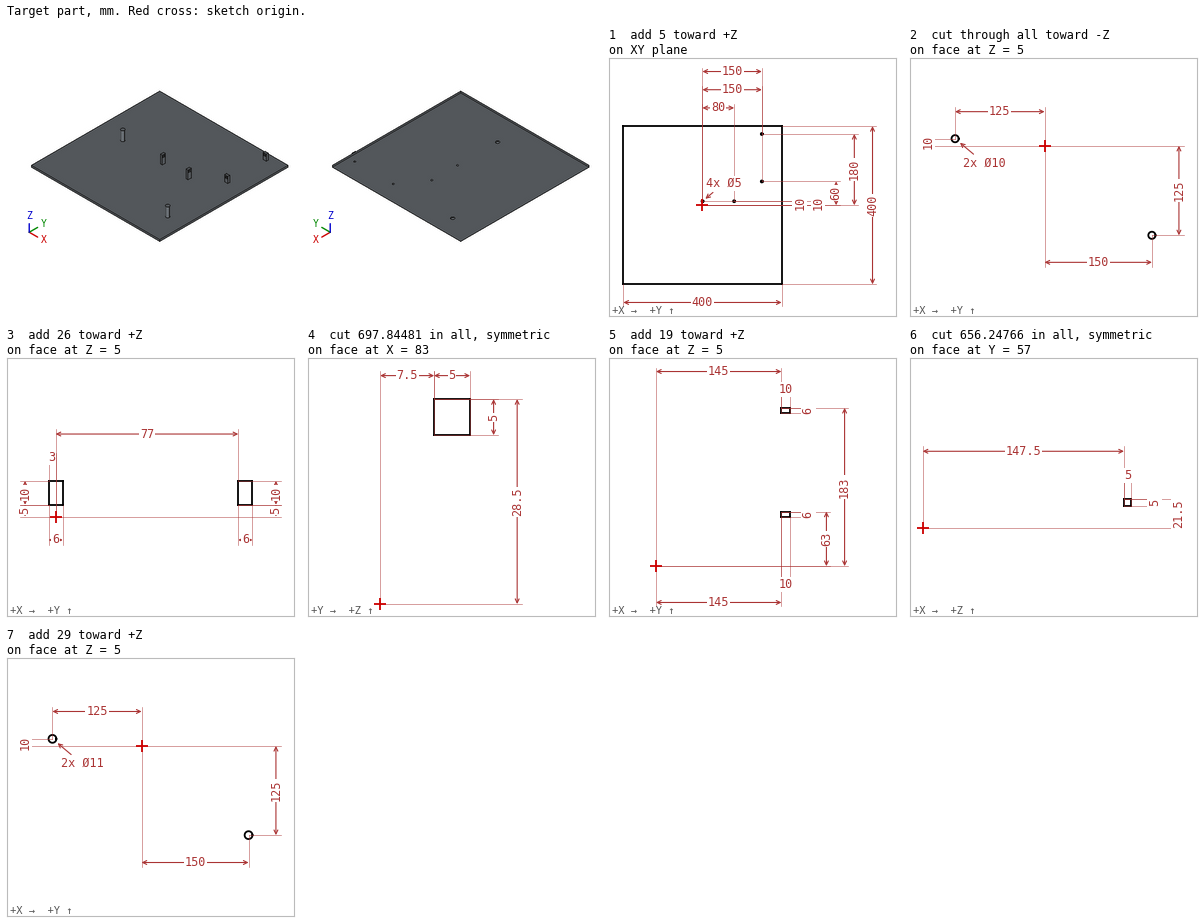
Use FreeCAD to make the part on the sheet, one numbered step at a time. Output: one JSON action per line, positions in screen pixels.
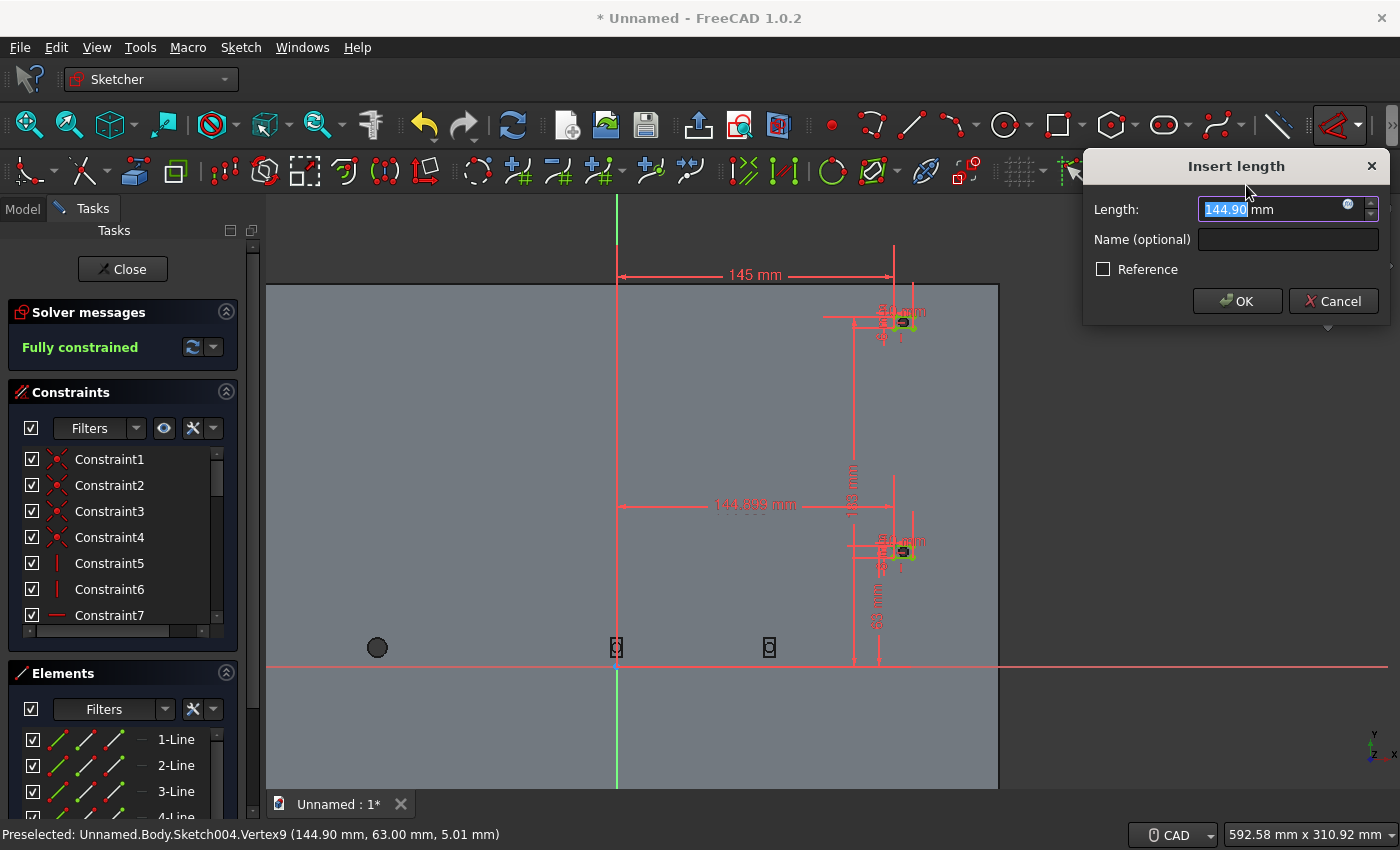
{"action": "type", "text": "145"}
{"action": "key", "text": "Return"}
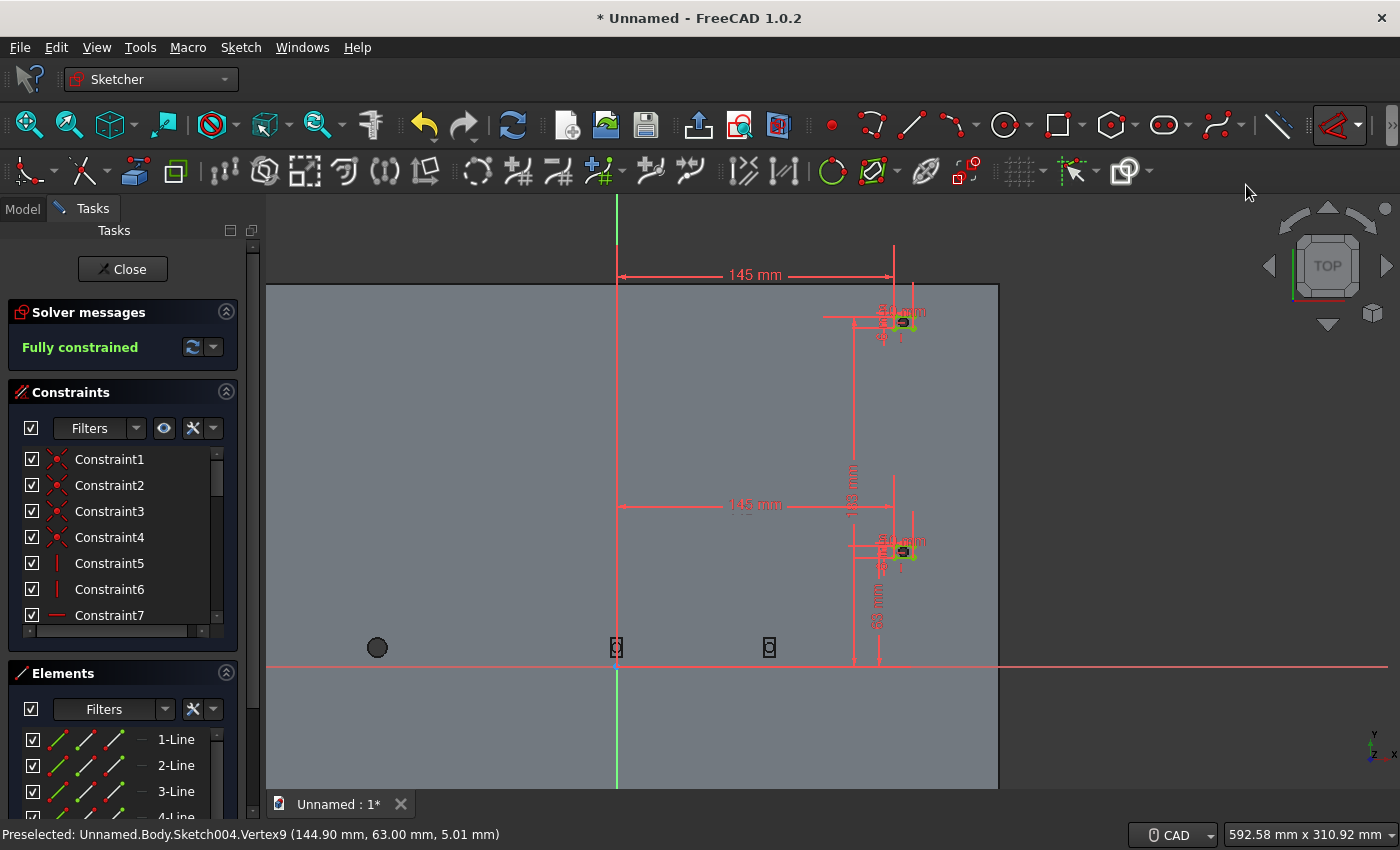
{"action": "left_click", "coordinate": [123, 269]}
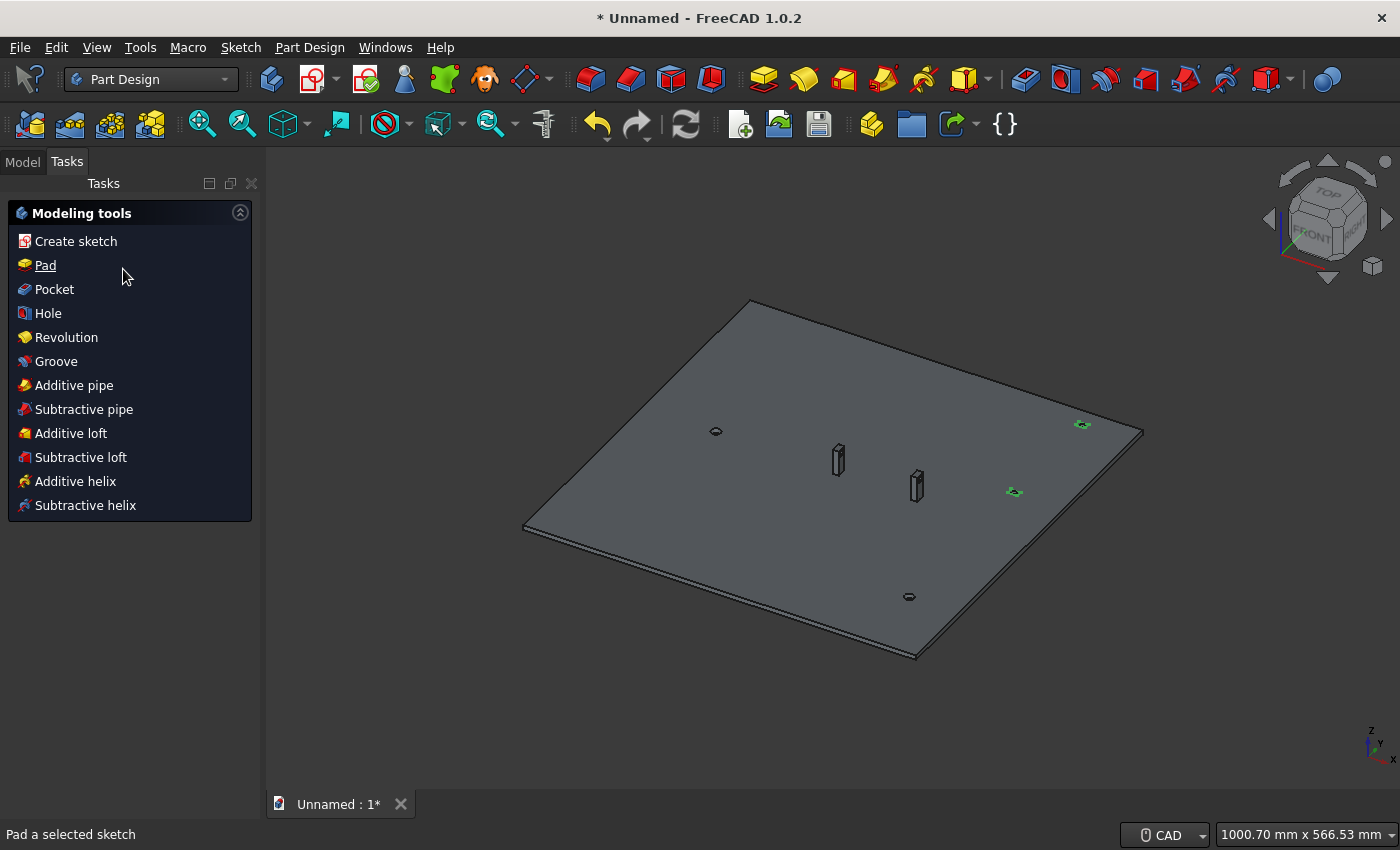
{"action": "left_click", "coordinate": [764, 80]}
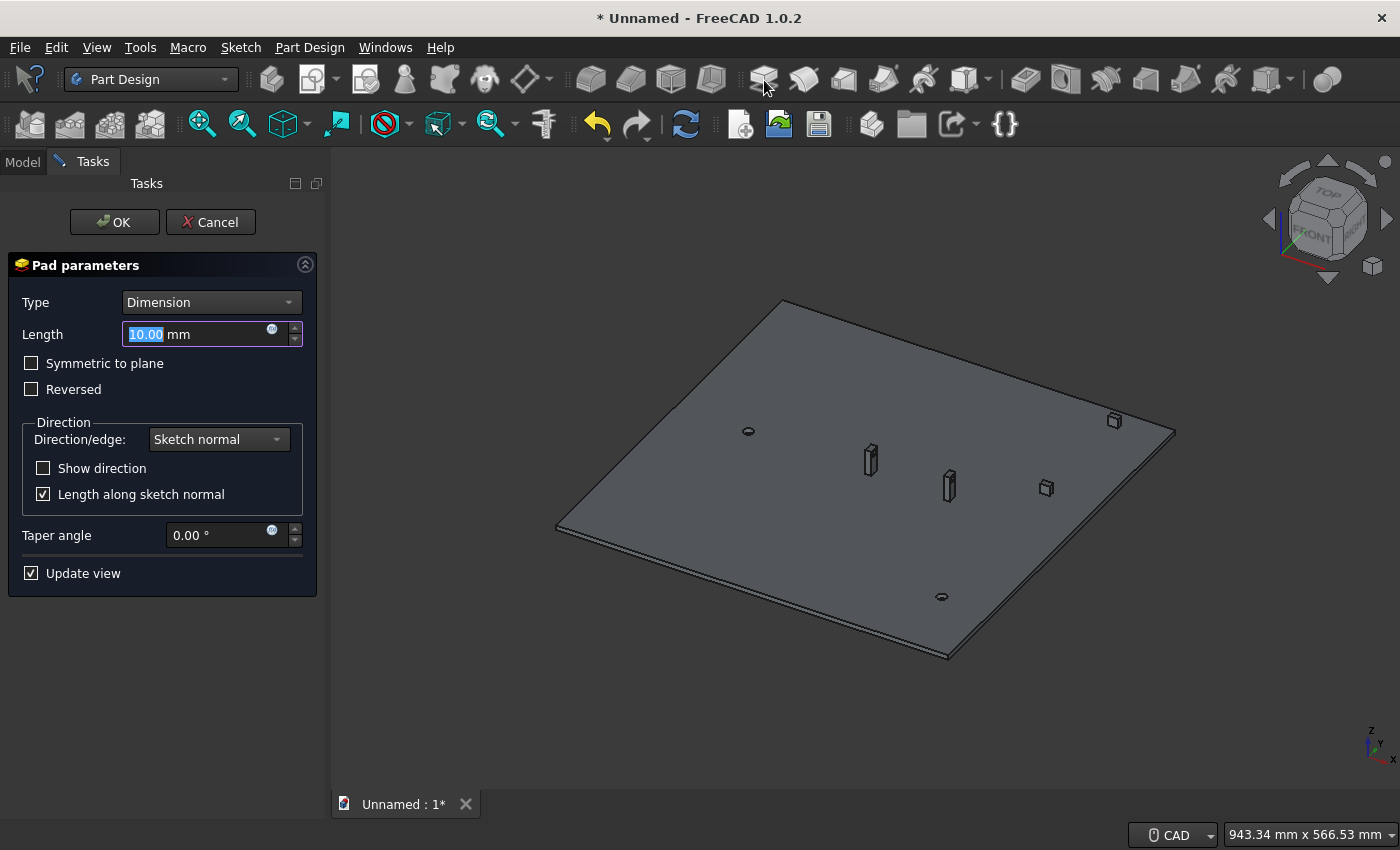
{"action": "type", "text": "19"}
{"action": "key", "text": "Tab"}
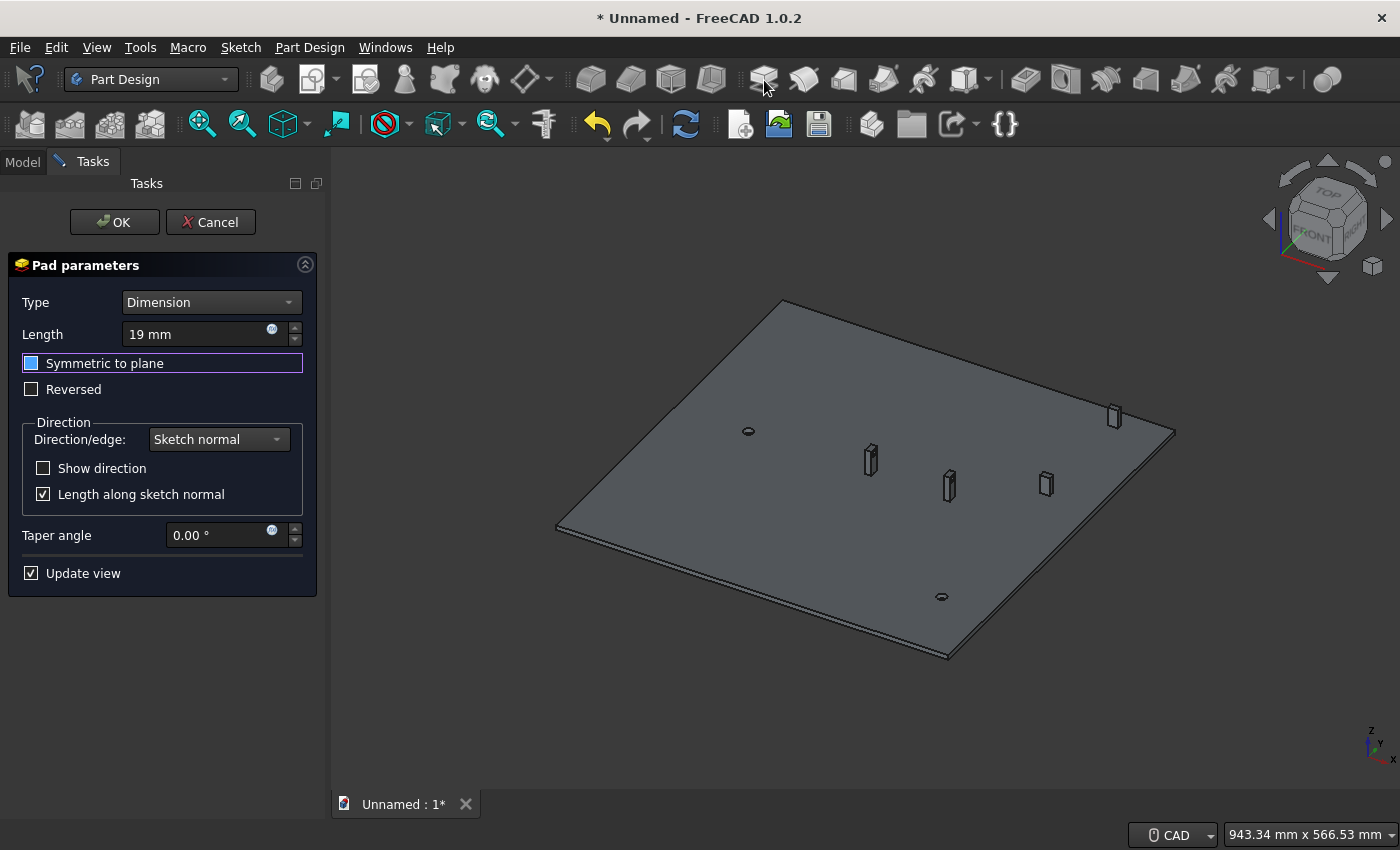
{"action": "left_click", "coordinate": [115, 222]}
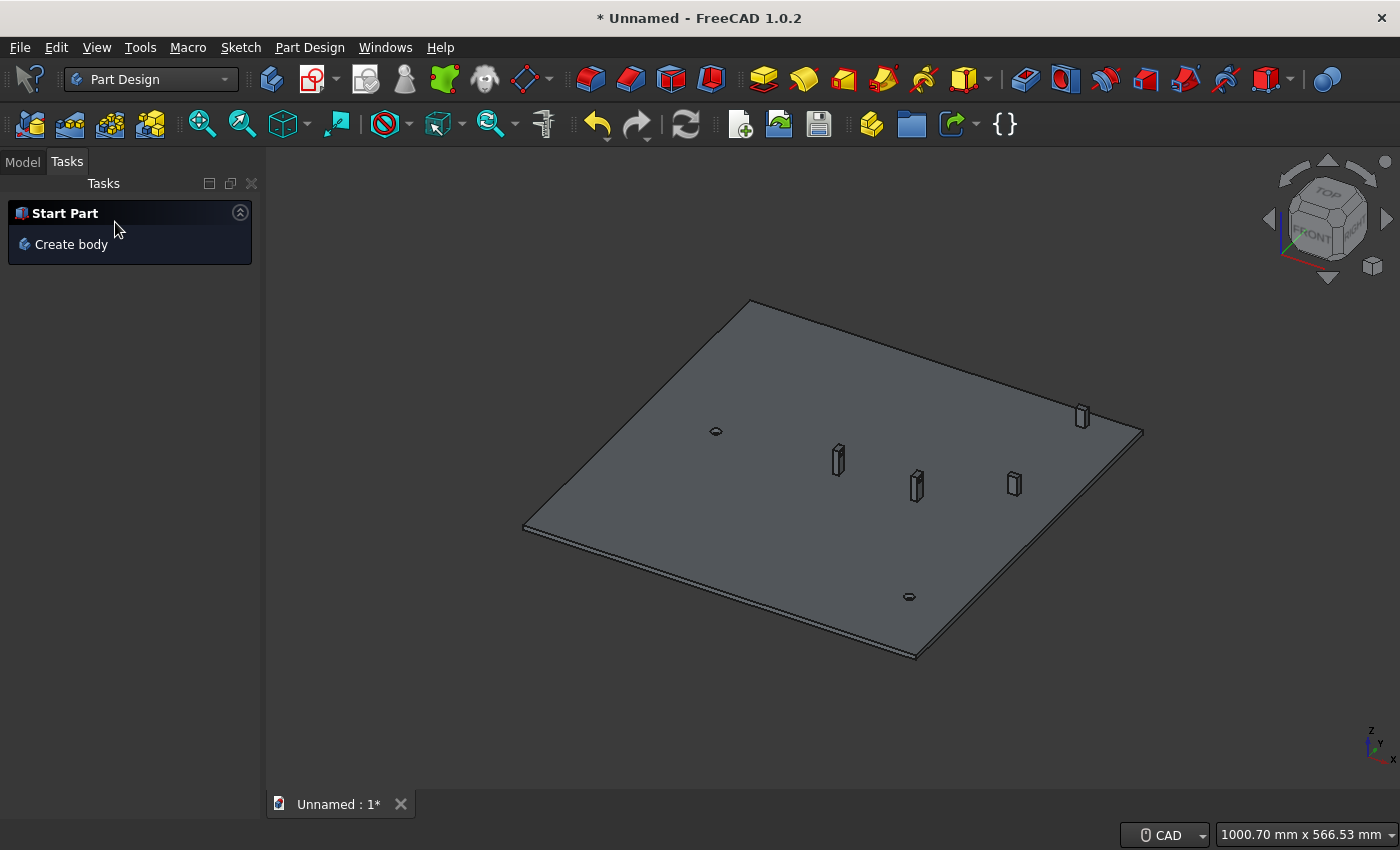
{"action": "scroll", "coordinate": [1013, 482], "scroll_direction": "up", "scroll_amount": 4}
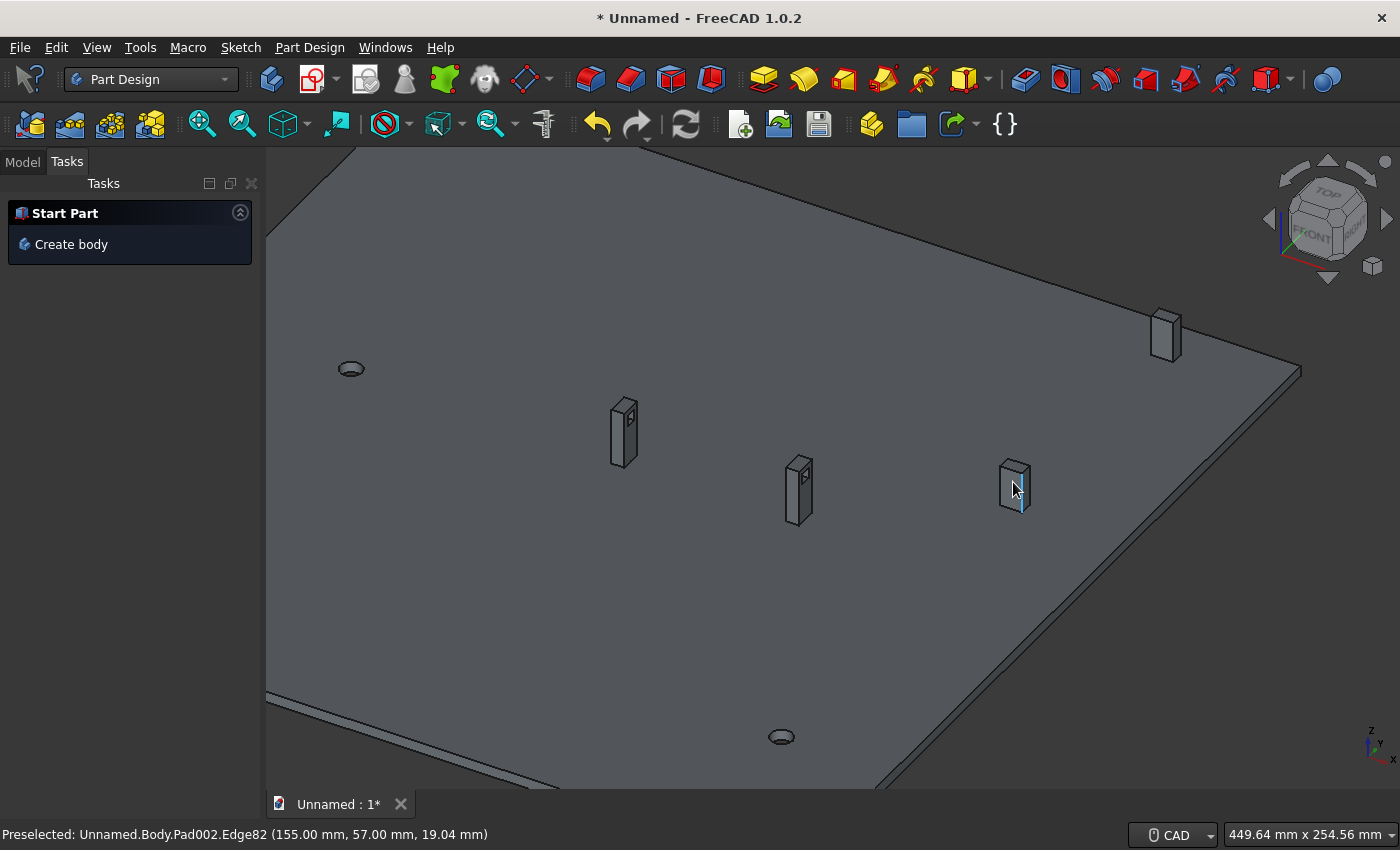
{"action": "left_click", "coordinate": [1011, 483]}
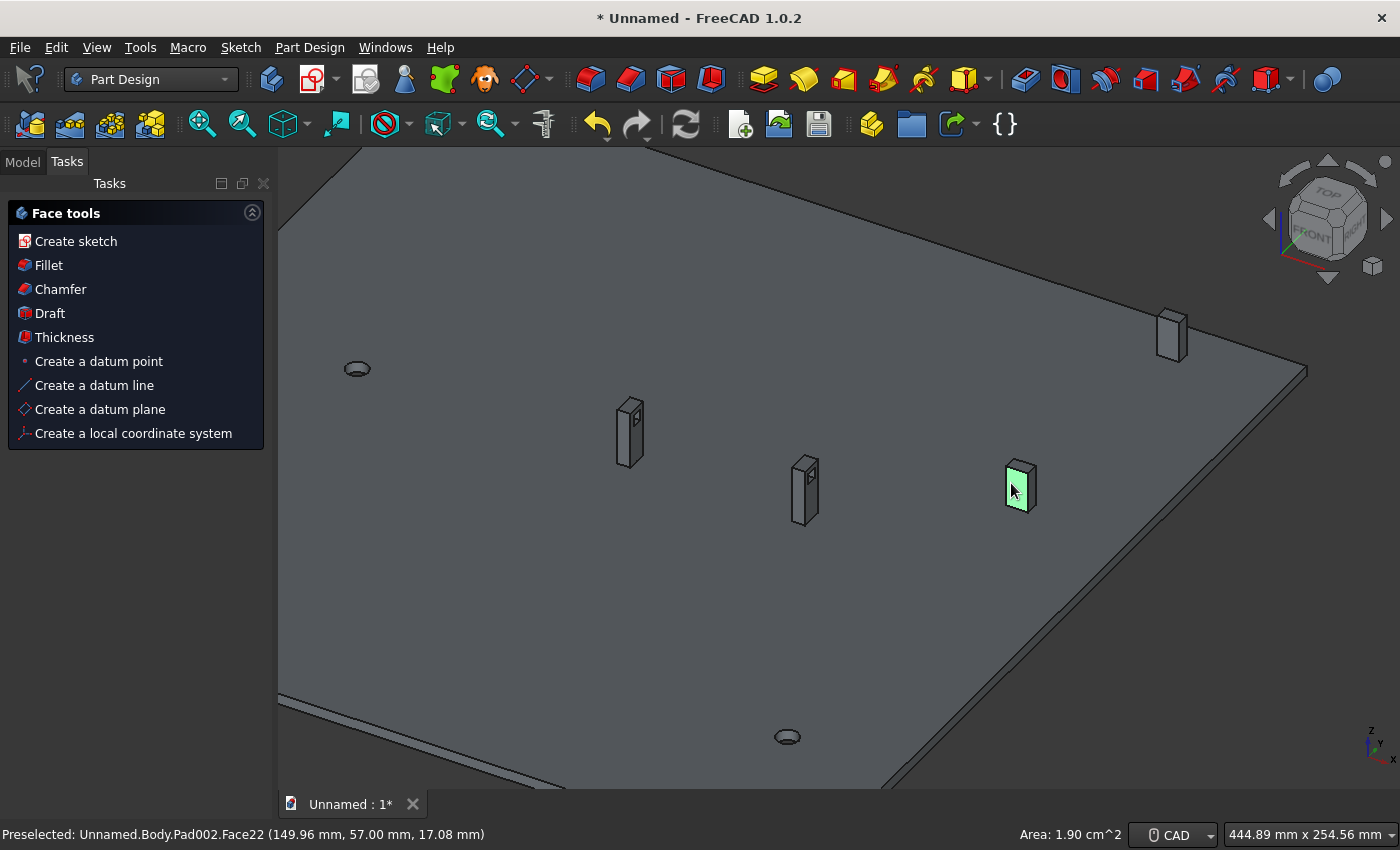
{"action": "left_click", "coordinate": [312, 80]}